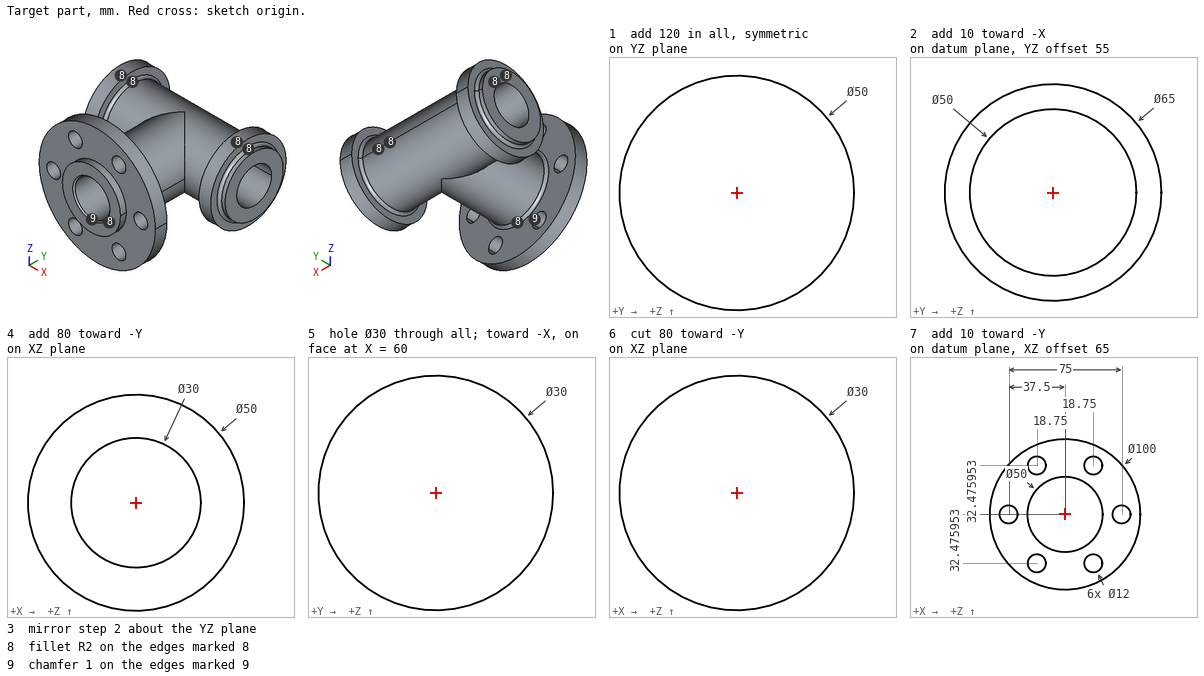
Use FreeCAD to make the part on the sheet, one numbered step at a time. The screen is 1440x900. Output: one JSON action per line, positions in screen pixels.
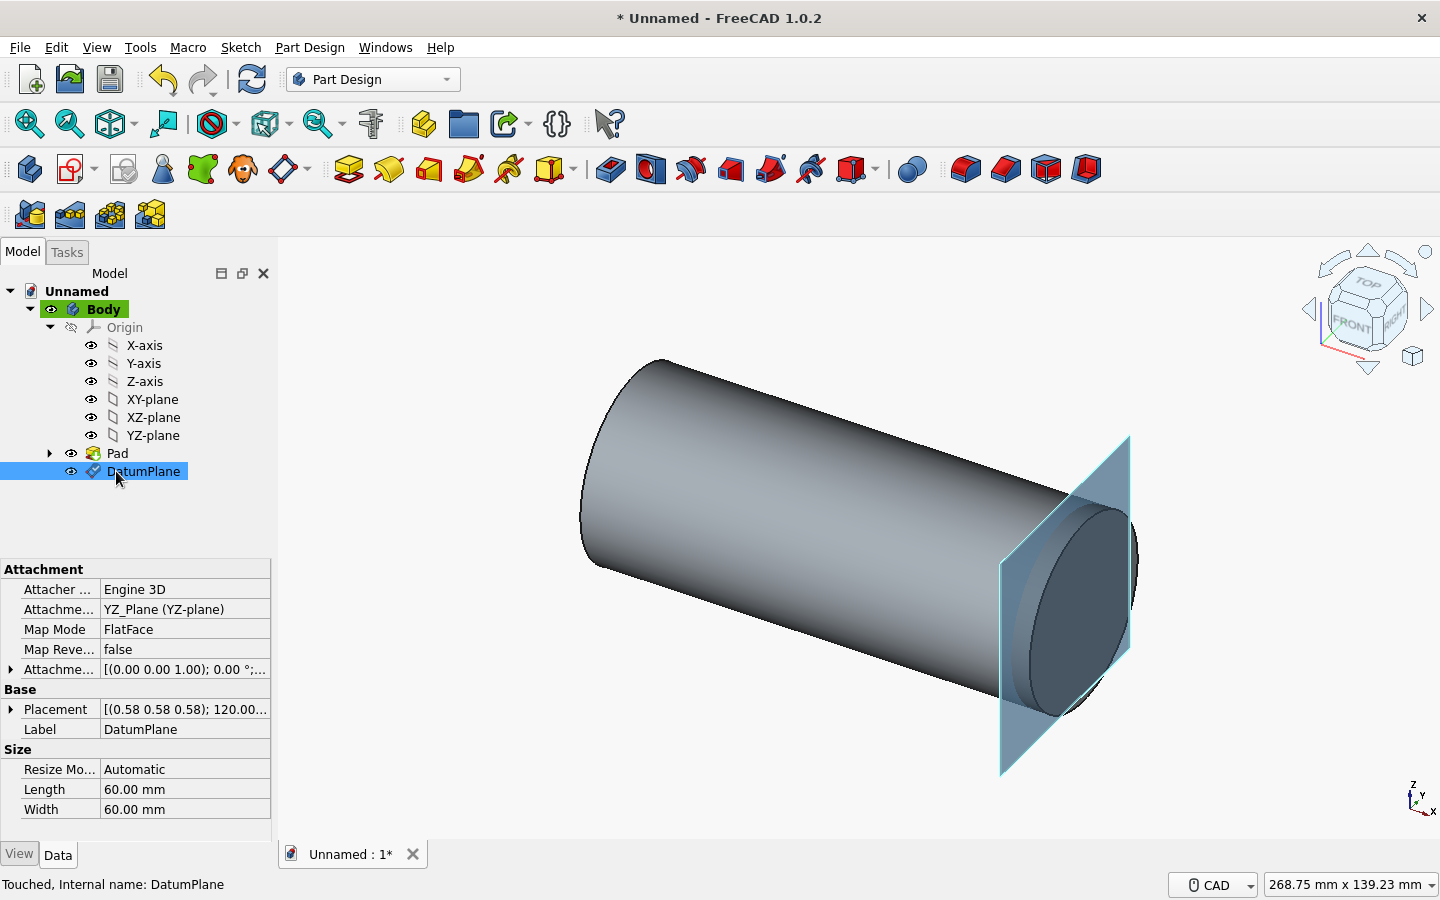
{"action": "left_click", "coordinate": [70, 170]}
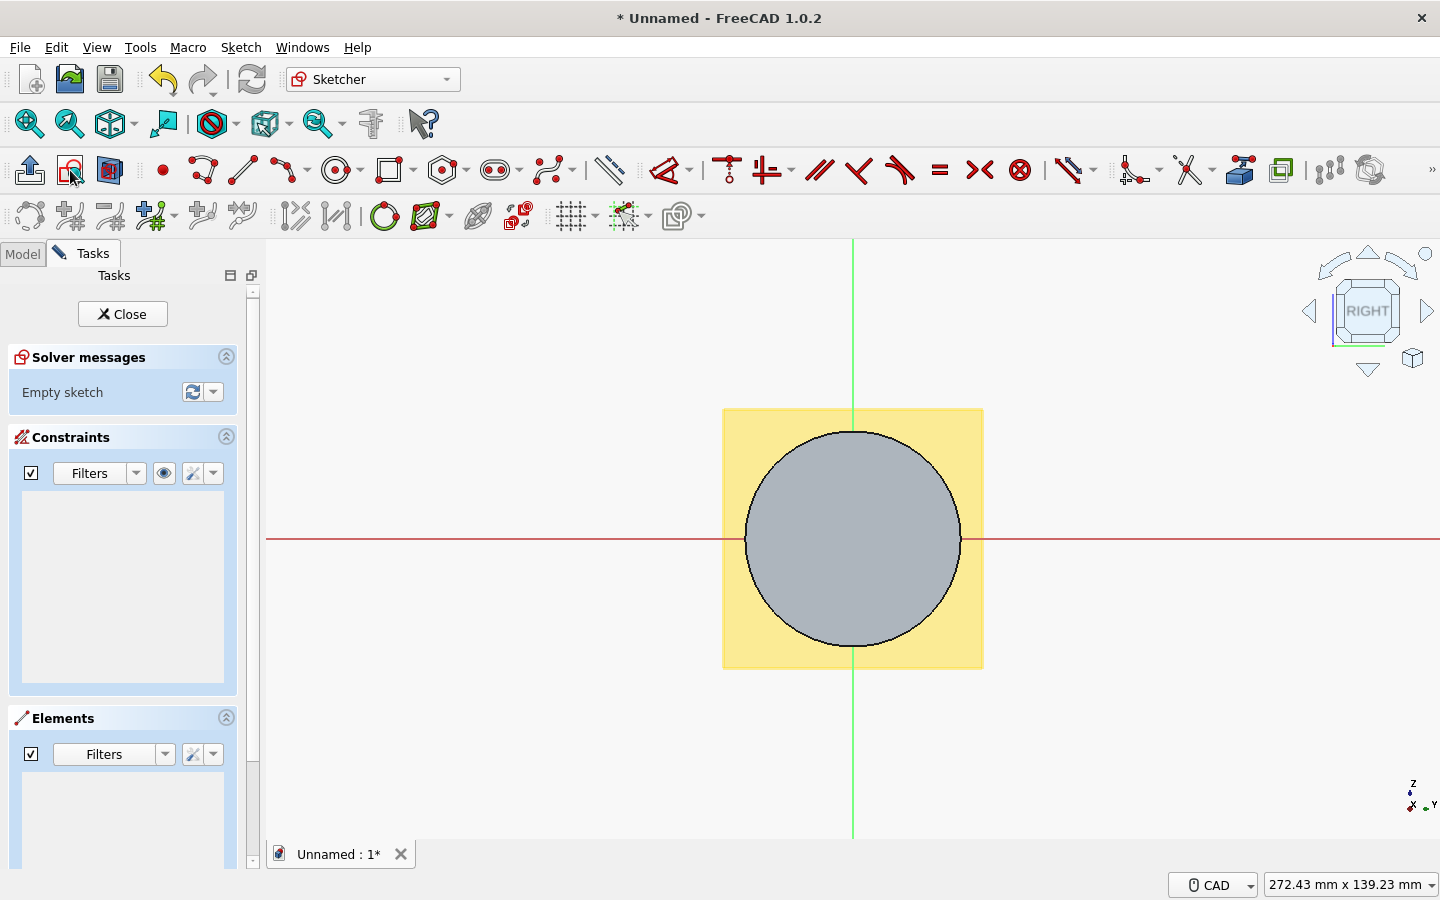
{"action": "key", "text": "q s"}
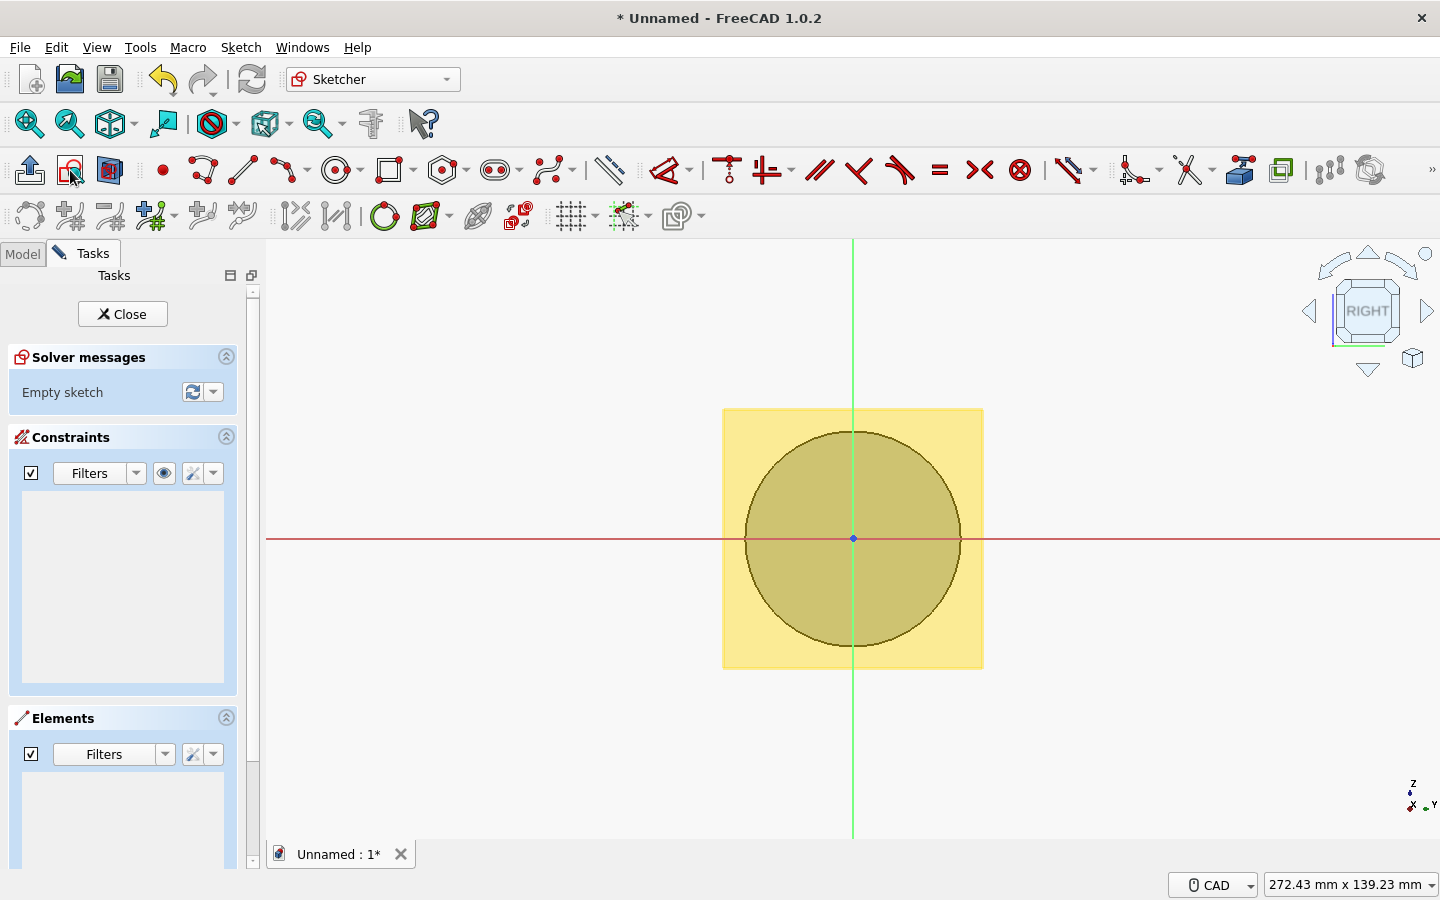
{"action": "scroll", "coordinate": [992, 539], "scroll_direction": "up", "scroll_amount": 2}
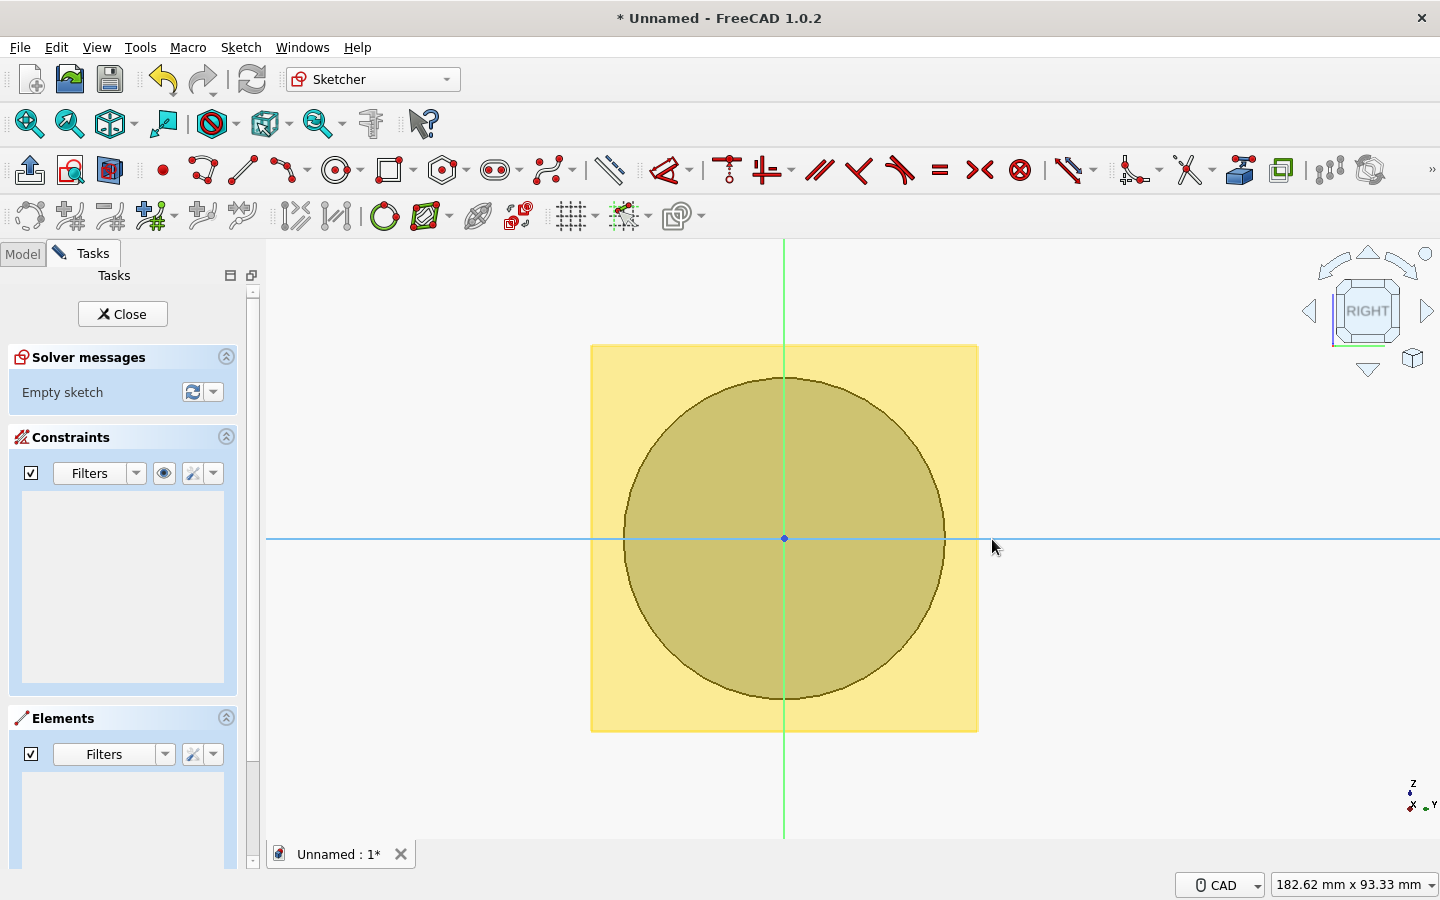
{"action": "left_click", "coordinate": [336, 170]}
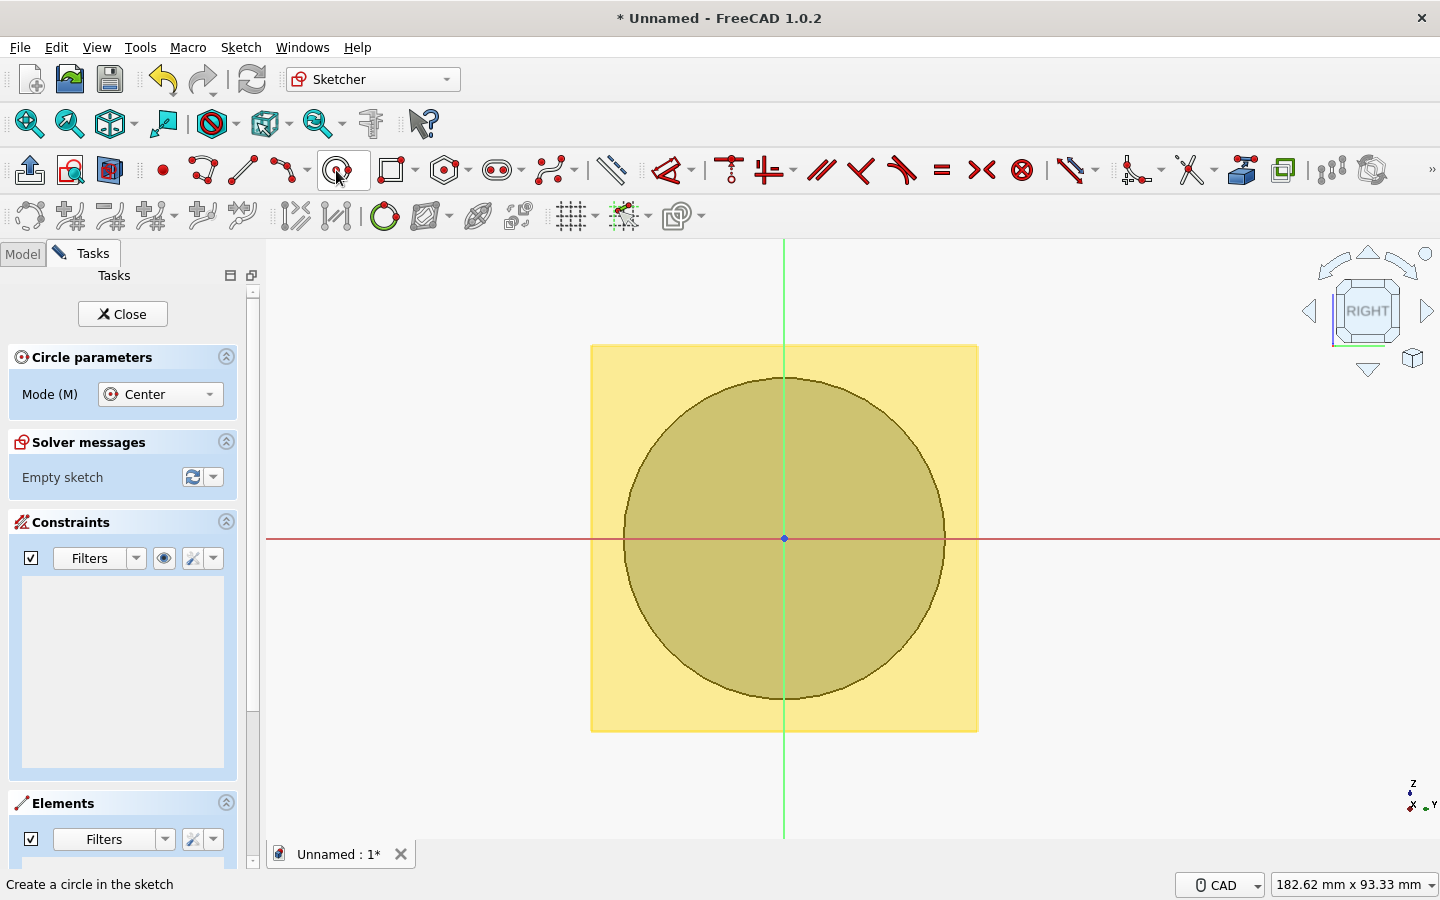
{"action": "left_click", "coordinate": [784, 539]}
{"action": "left_click", "coordinate": [932, 391]}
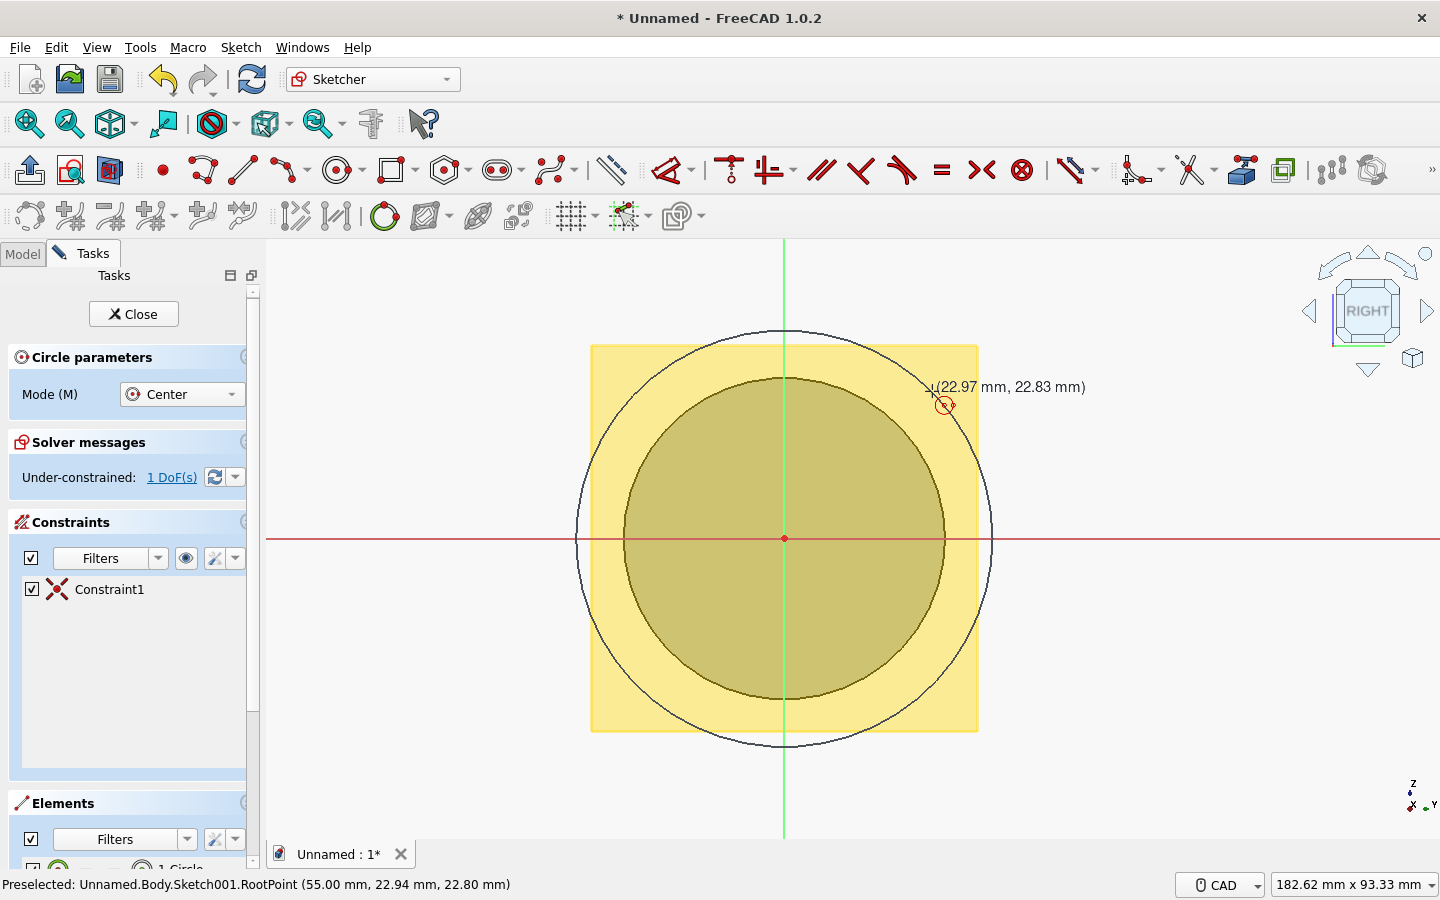
{"action": "left_click", "coordinate": [784, 539]}
{"action": "left_click", "coordinate": [898, 425]}
{"action": "key", "text": "Escape"}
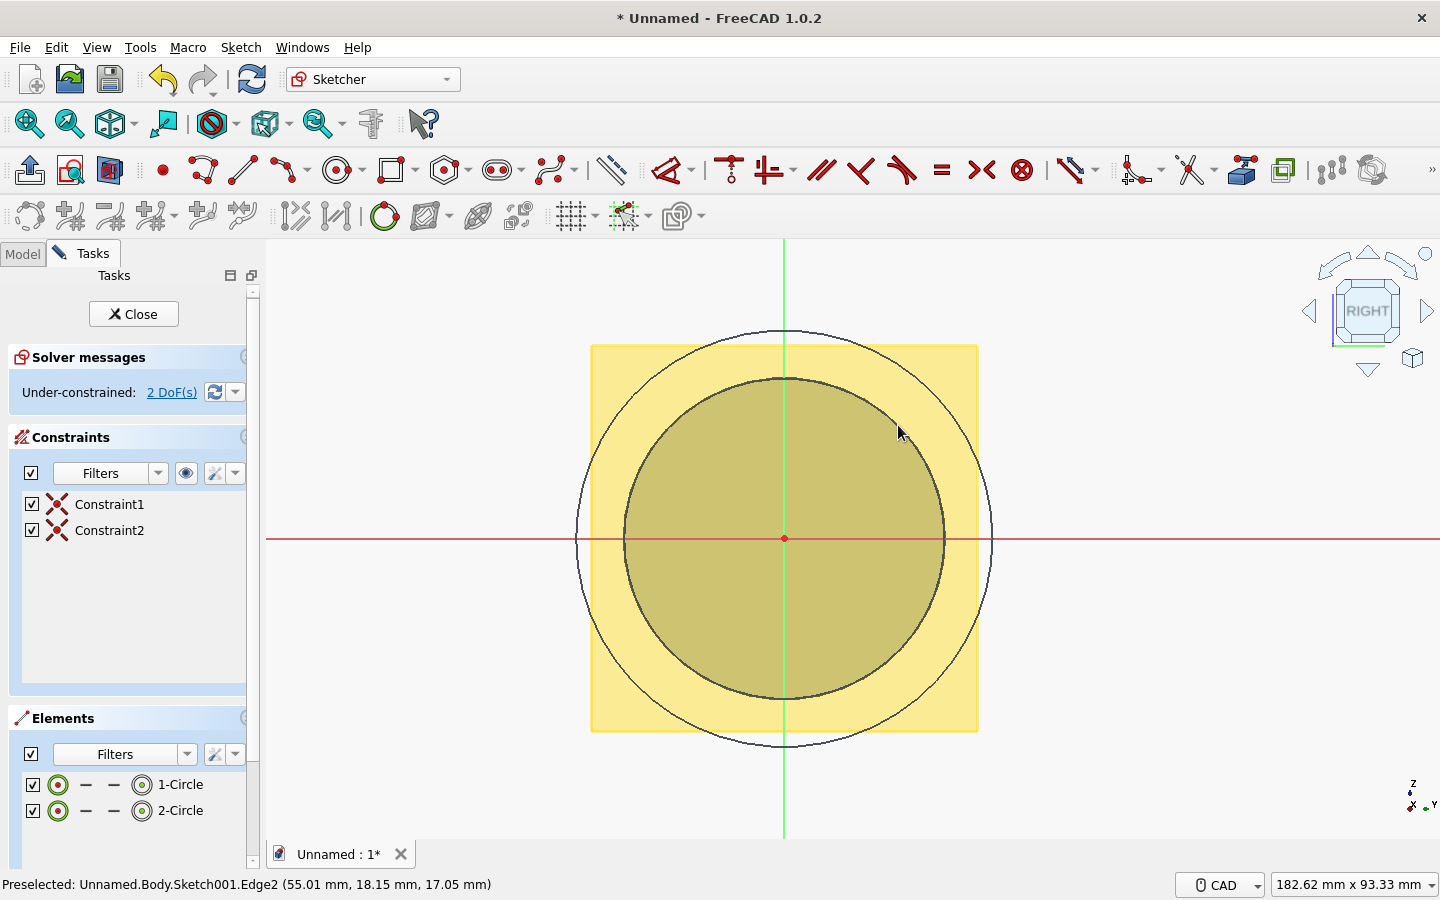
{"action": "left_click", "coordinate": [931, 391]}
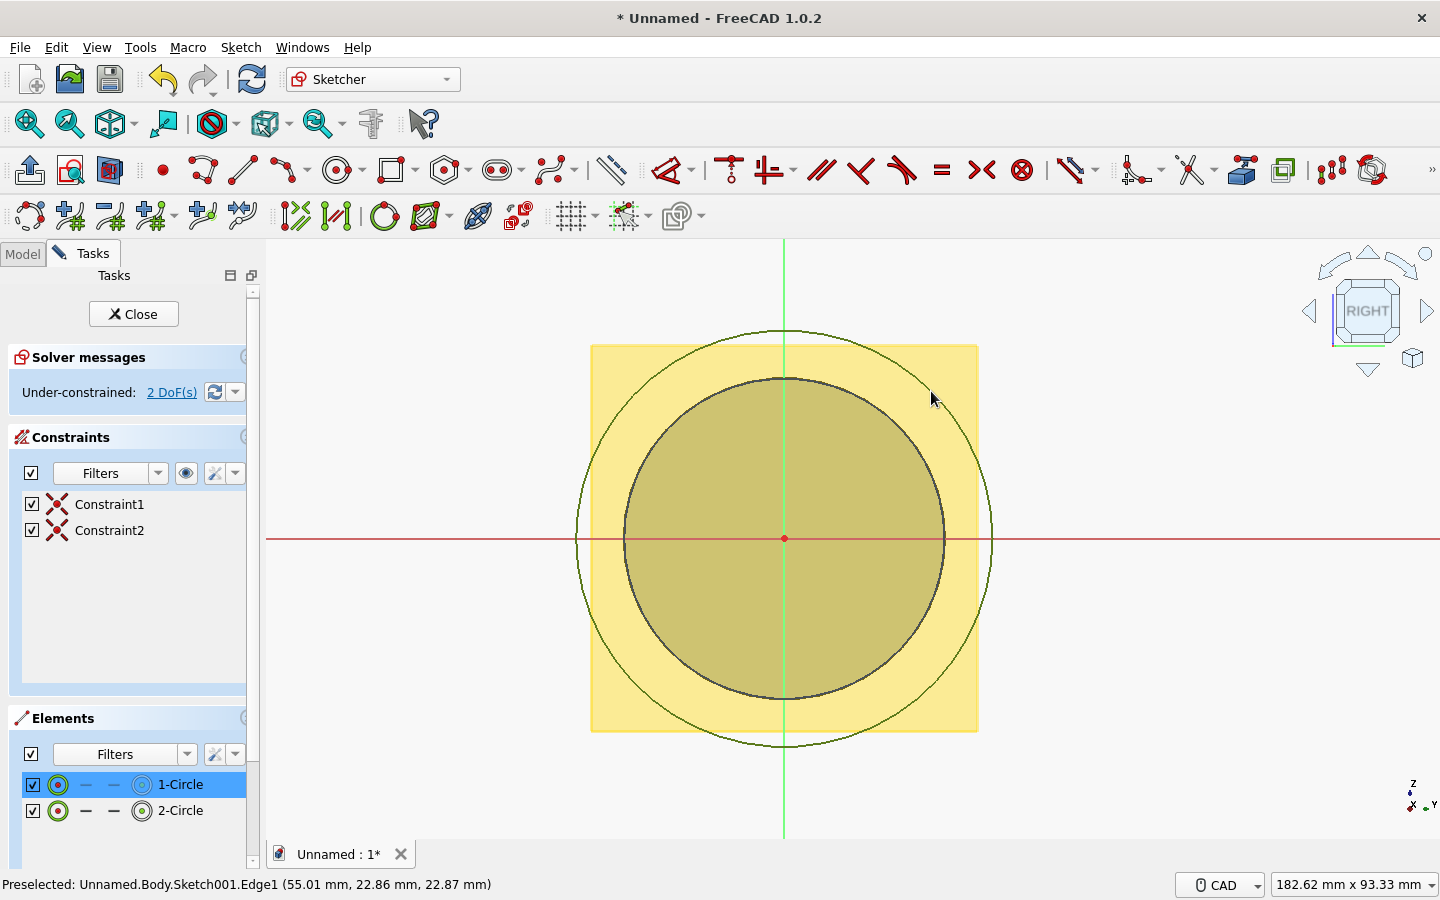
{"action": "key", "text": "k o"}